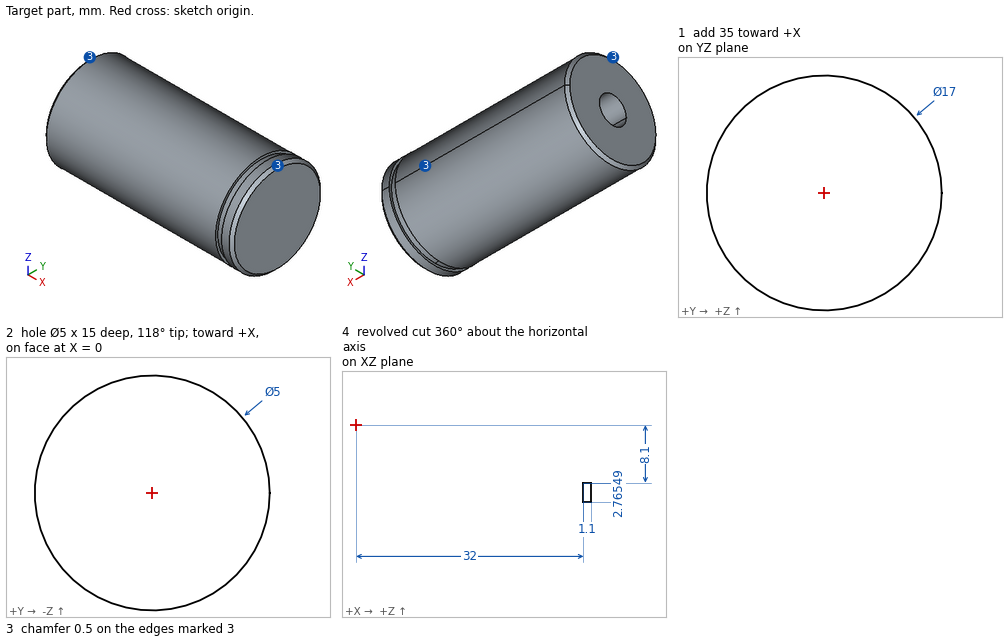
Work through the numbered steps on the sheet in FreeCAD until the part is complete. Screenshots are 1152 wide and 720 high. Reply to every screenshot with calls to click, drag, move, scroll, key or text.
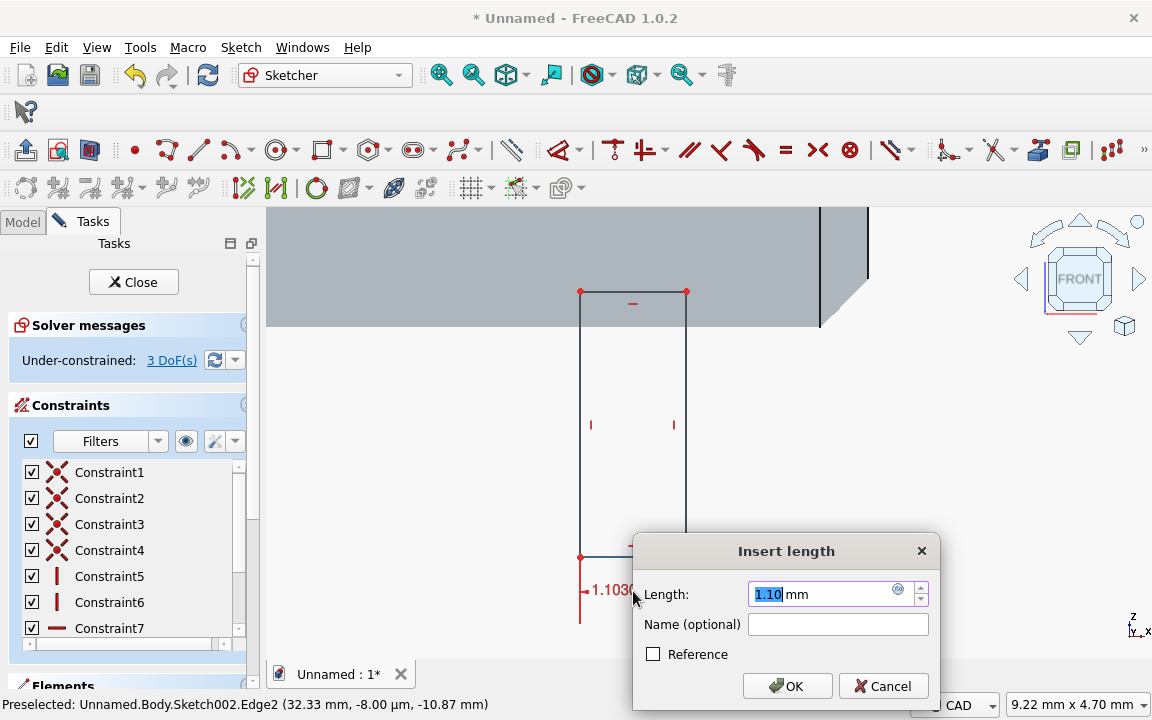
text(1.1)
key(Return)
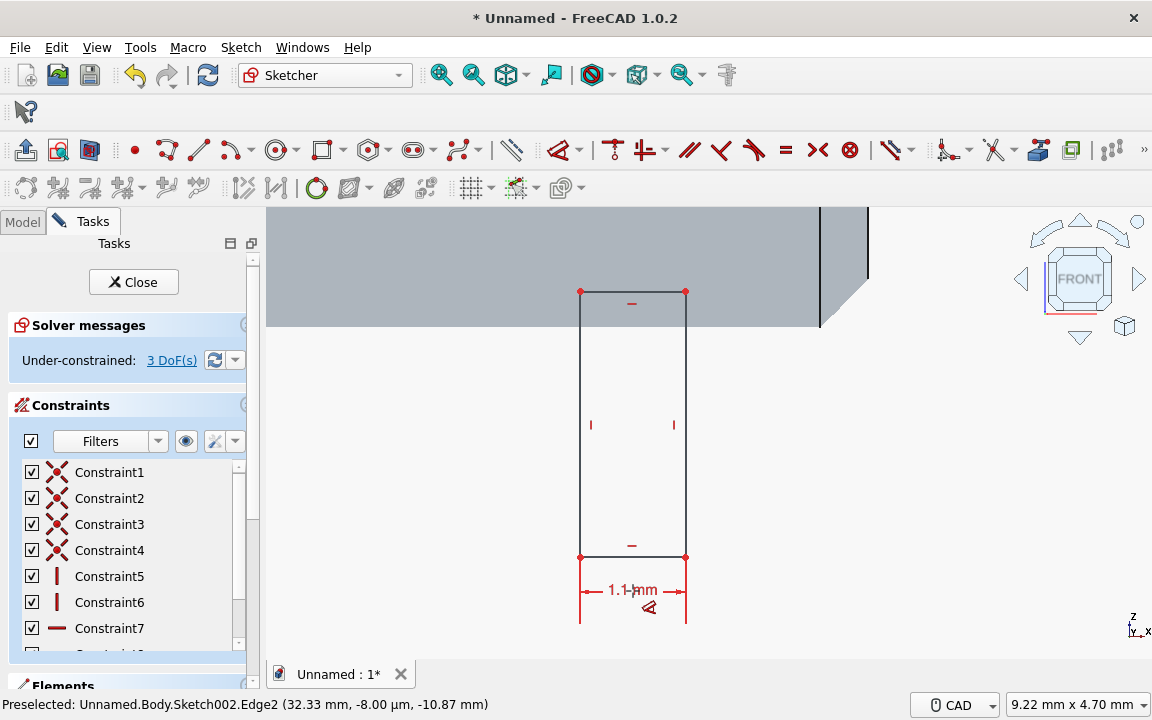
click(580, 292)
click(437, 326)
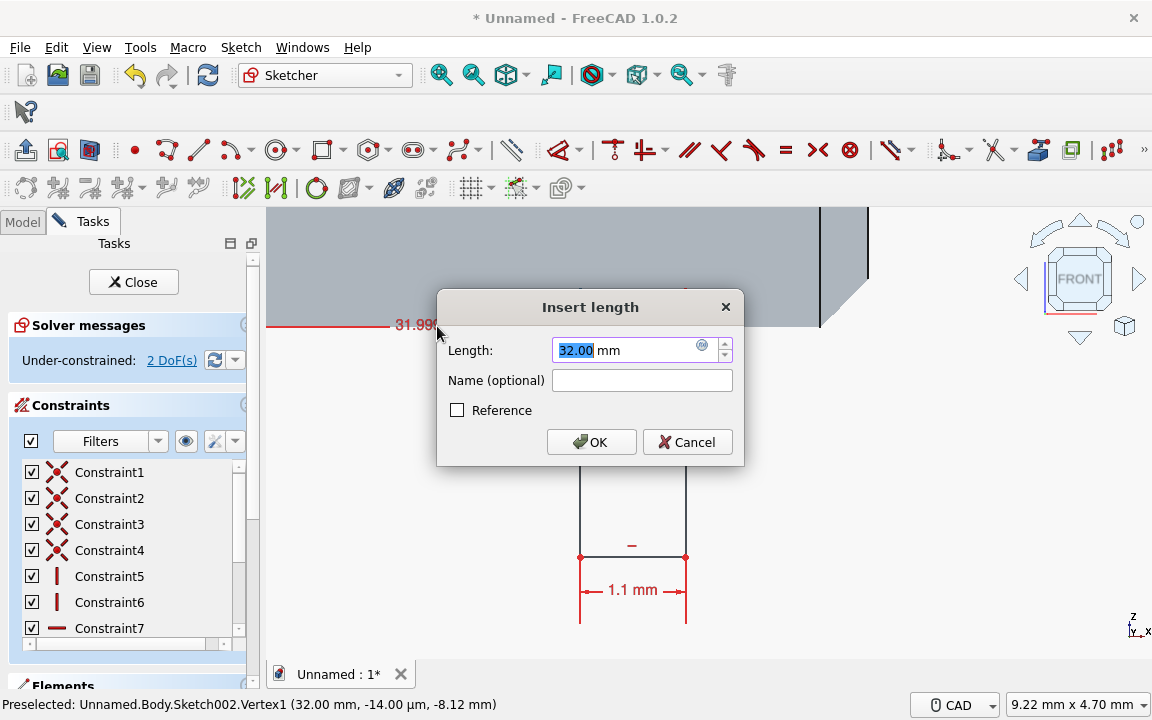
text(32)
key(Return)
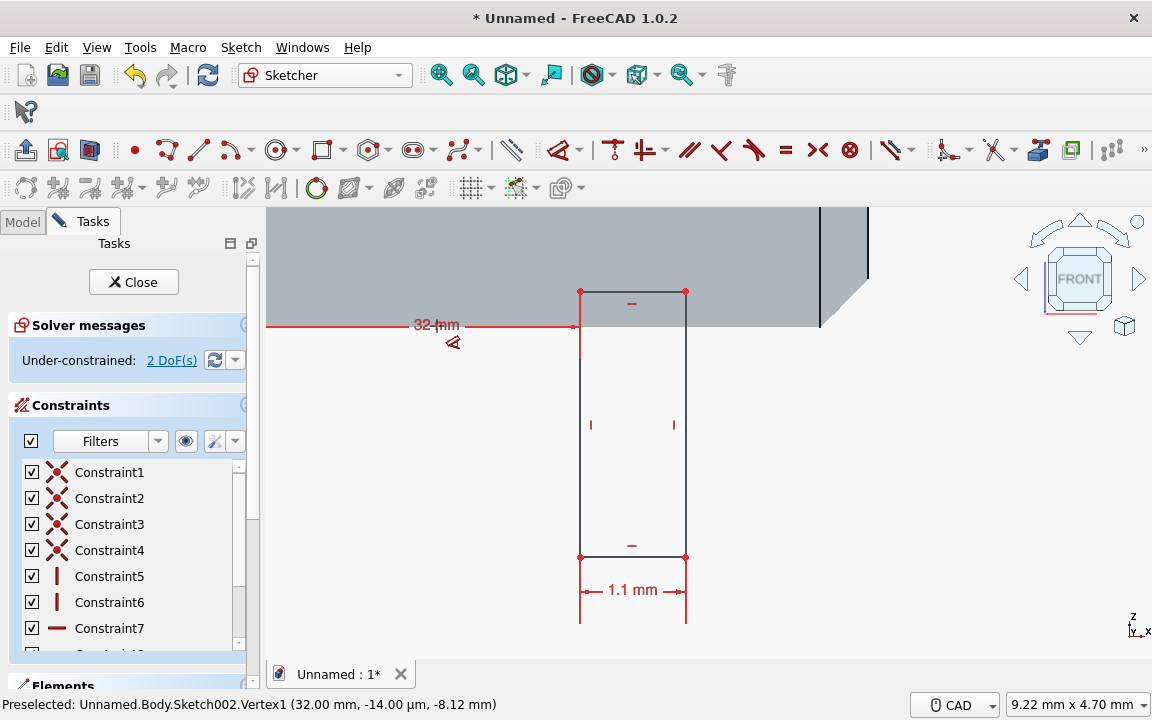
click(580, 292)
click(614, 263)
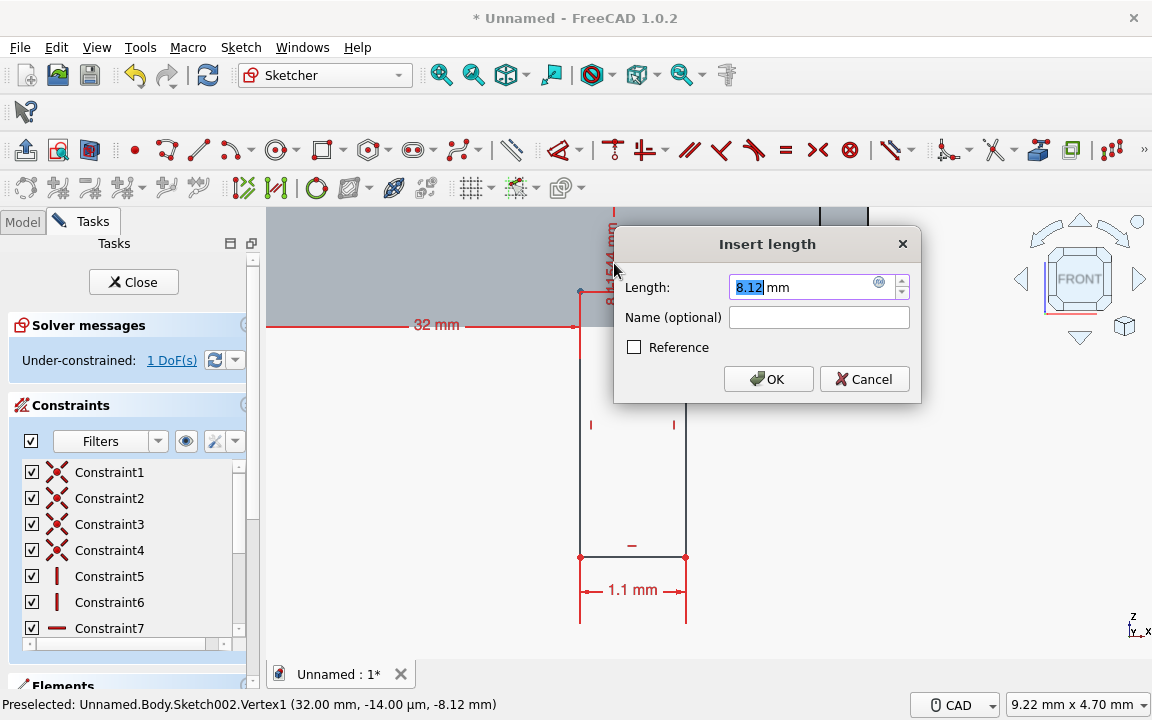
text(8.1)
key(Return)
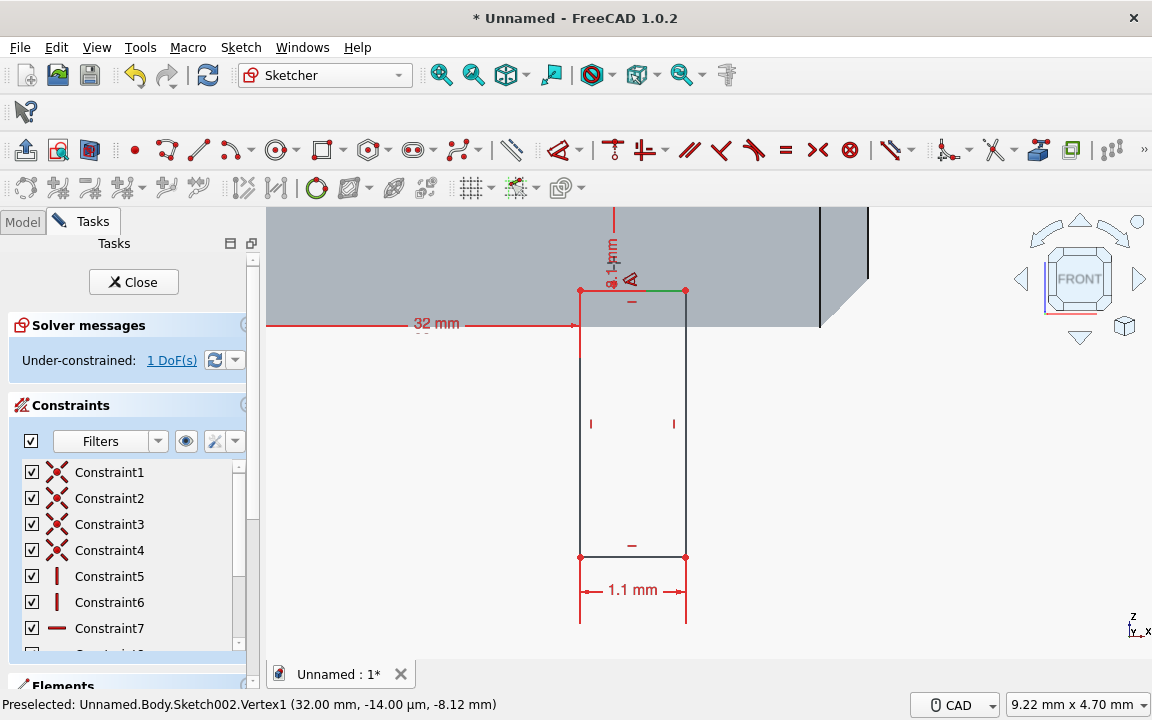
click(580, 370)
click(546, 424)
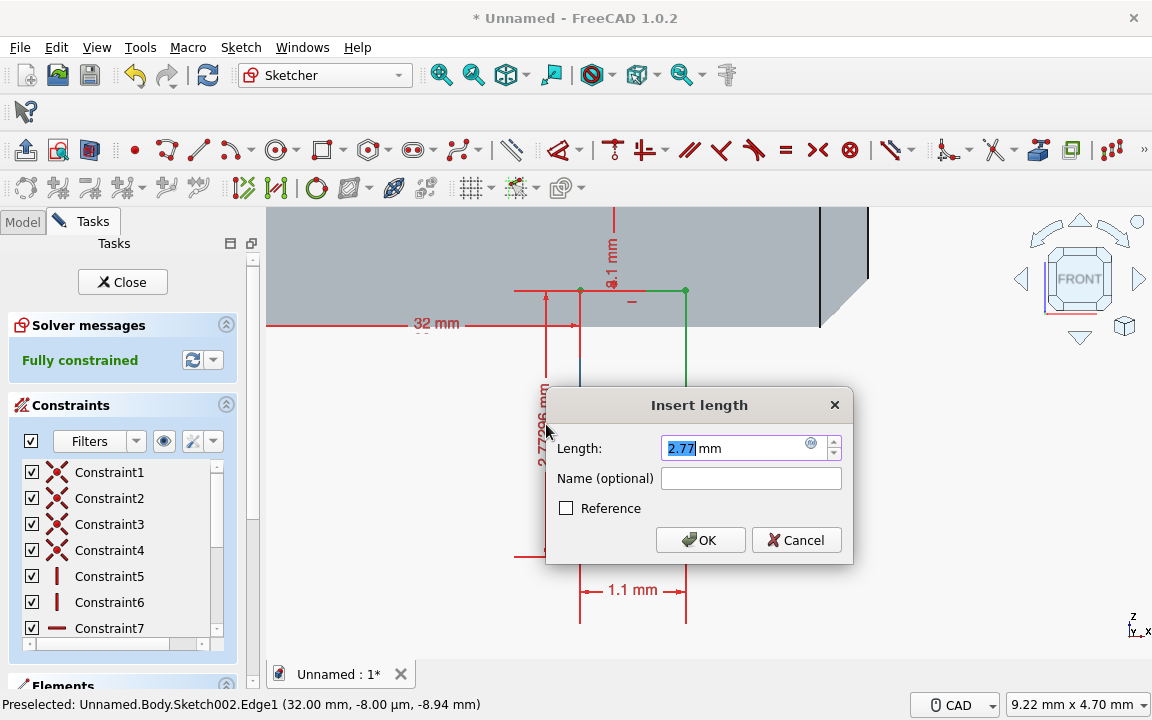
text(2.76549)
key(Return)
key(Escape)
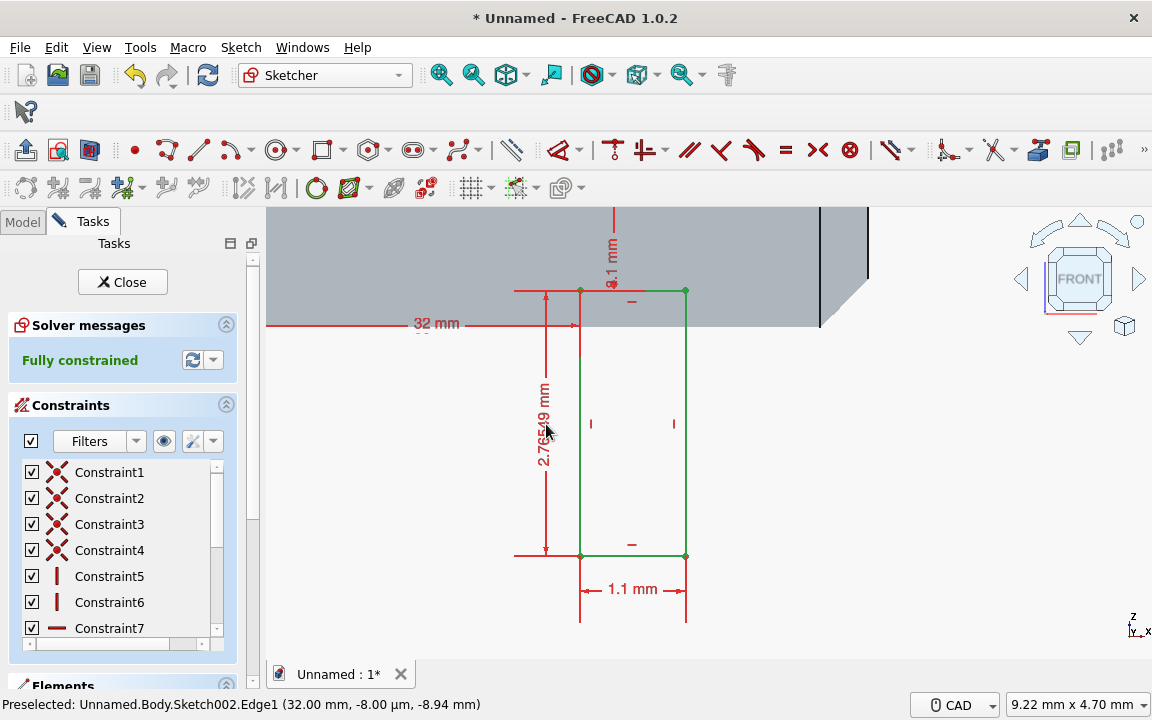
click(123, 282)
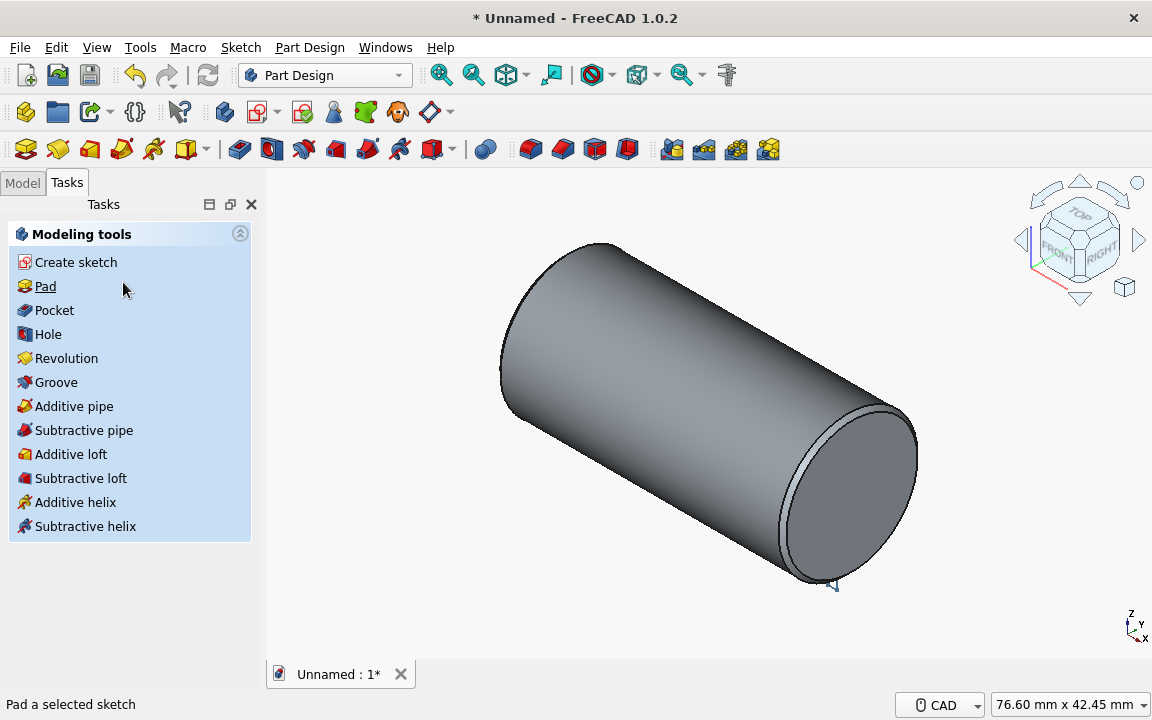
click(304, 150)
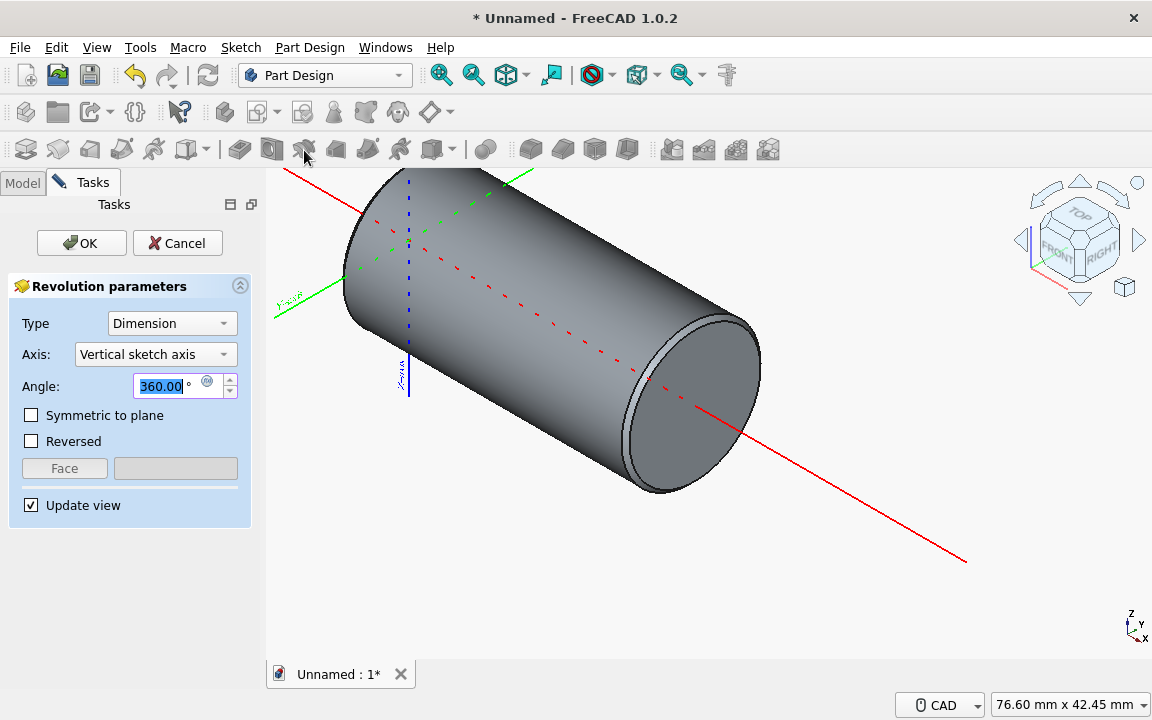
click(156, 354)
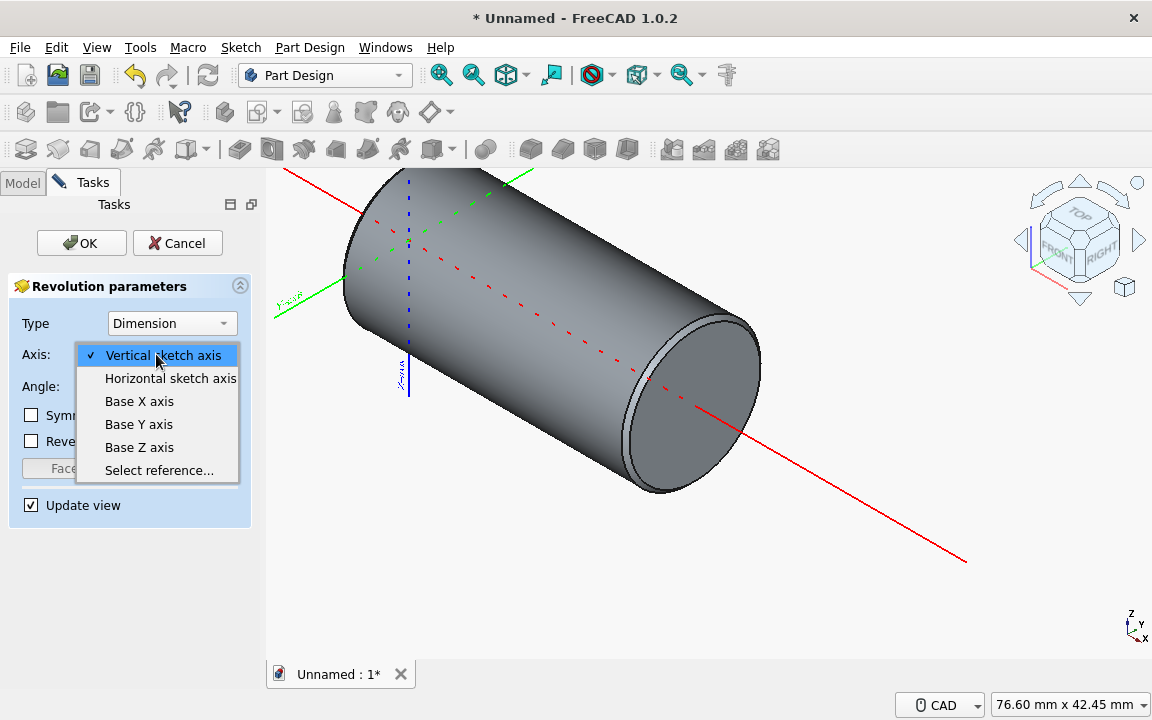
click(156, 378)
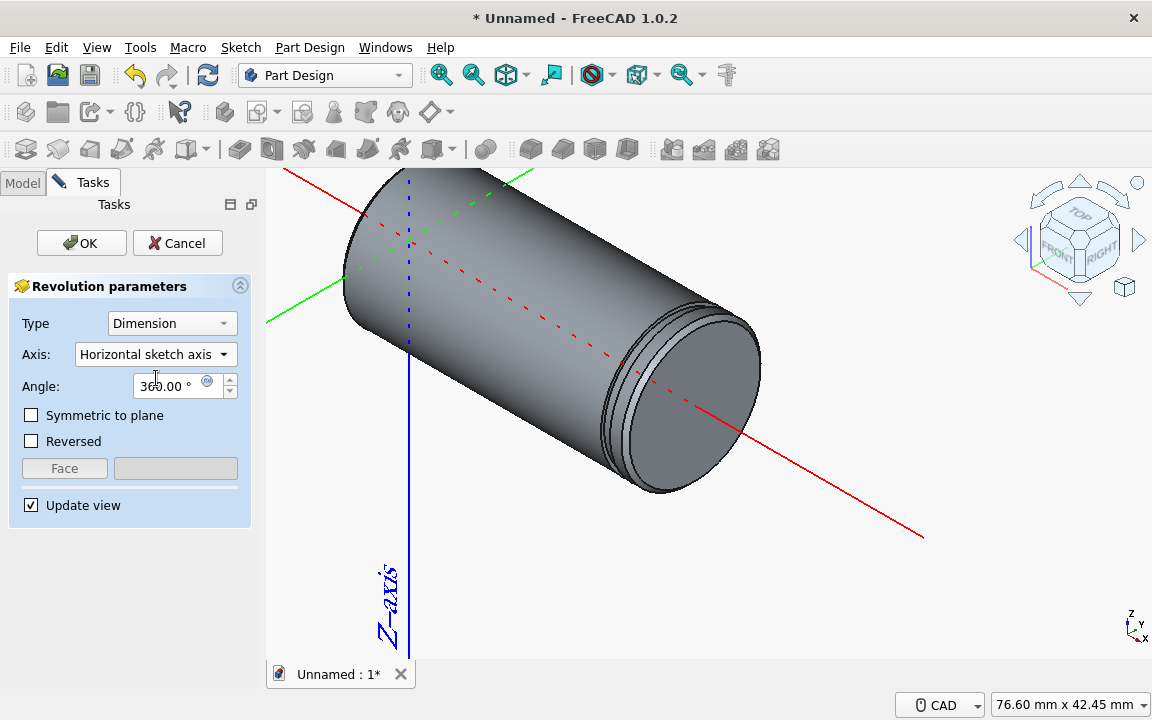
click(82, 243)